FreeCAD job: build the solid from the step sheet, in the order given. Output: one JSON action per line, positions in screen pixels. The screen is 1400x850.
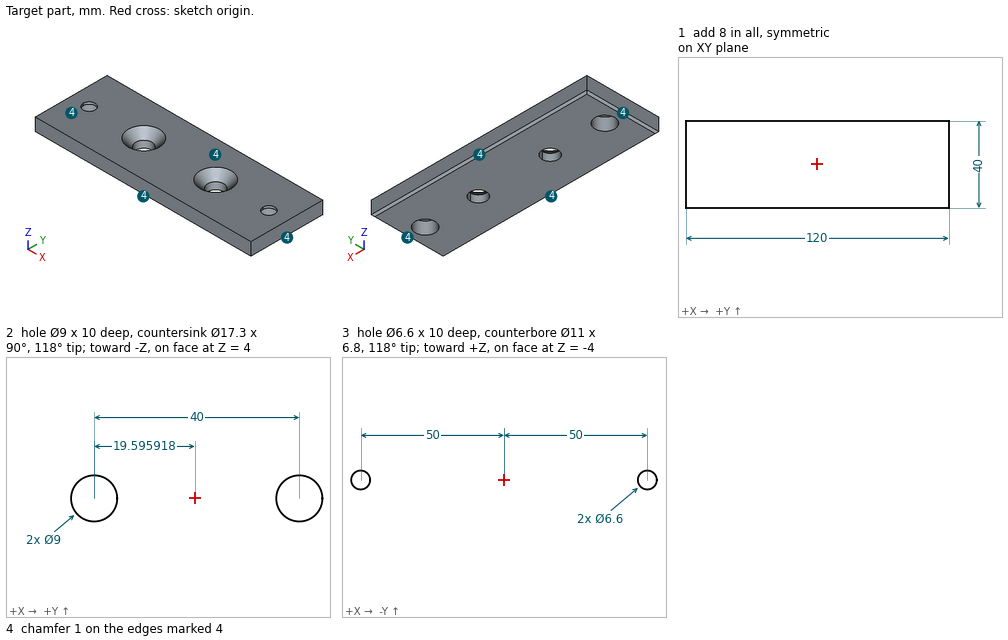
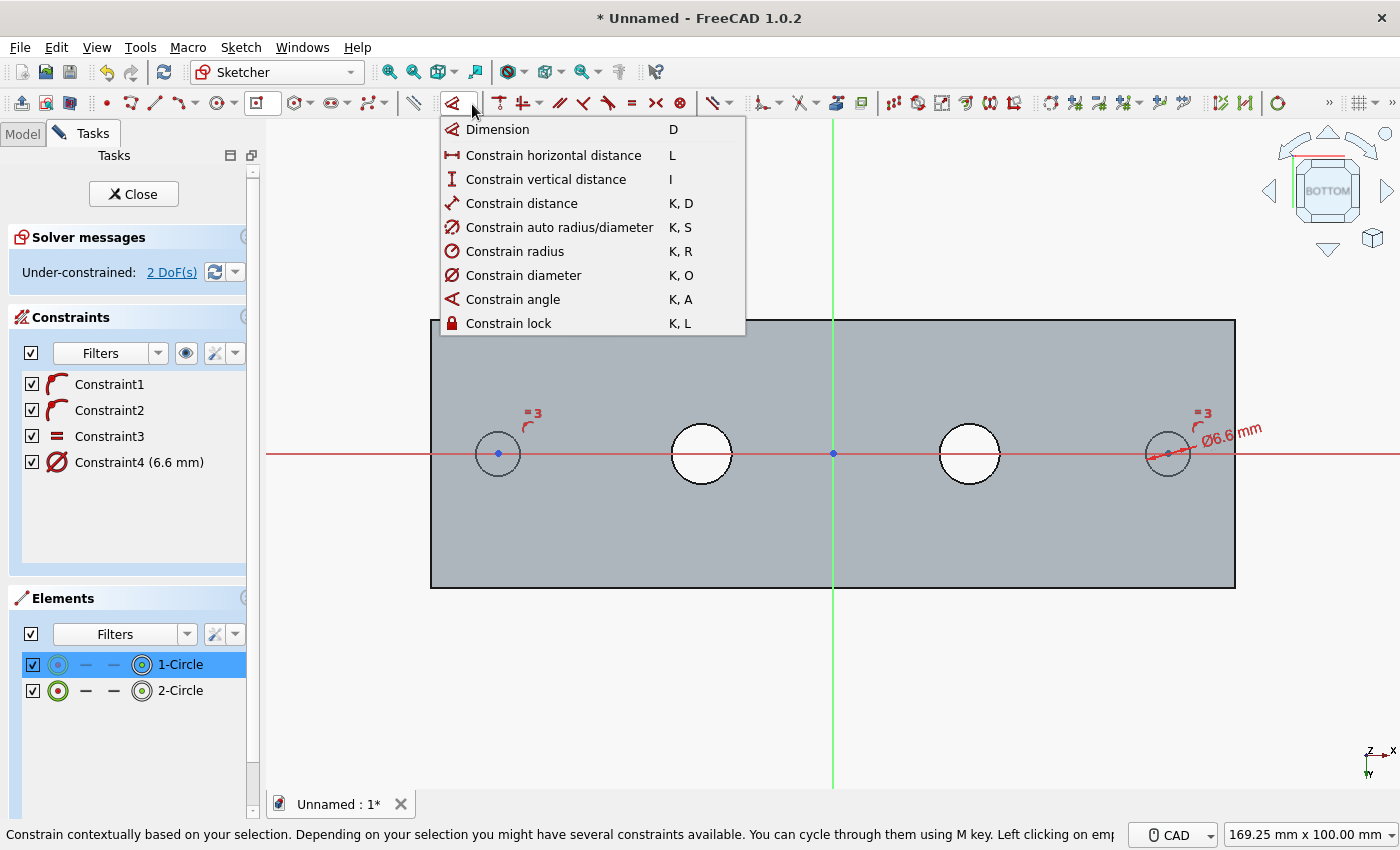
{"action": "left_click", "coordinate": [593, 155]}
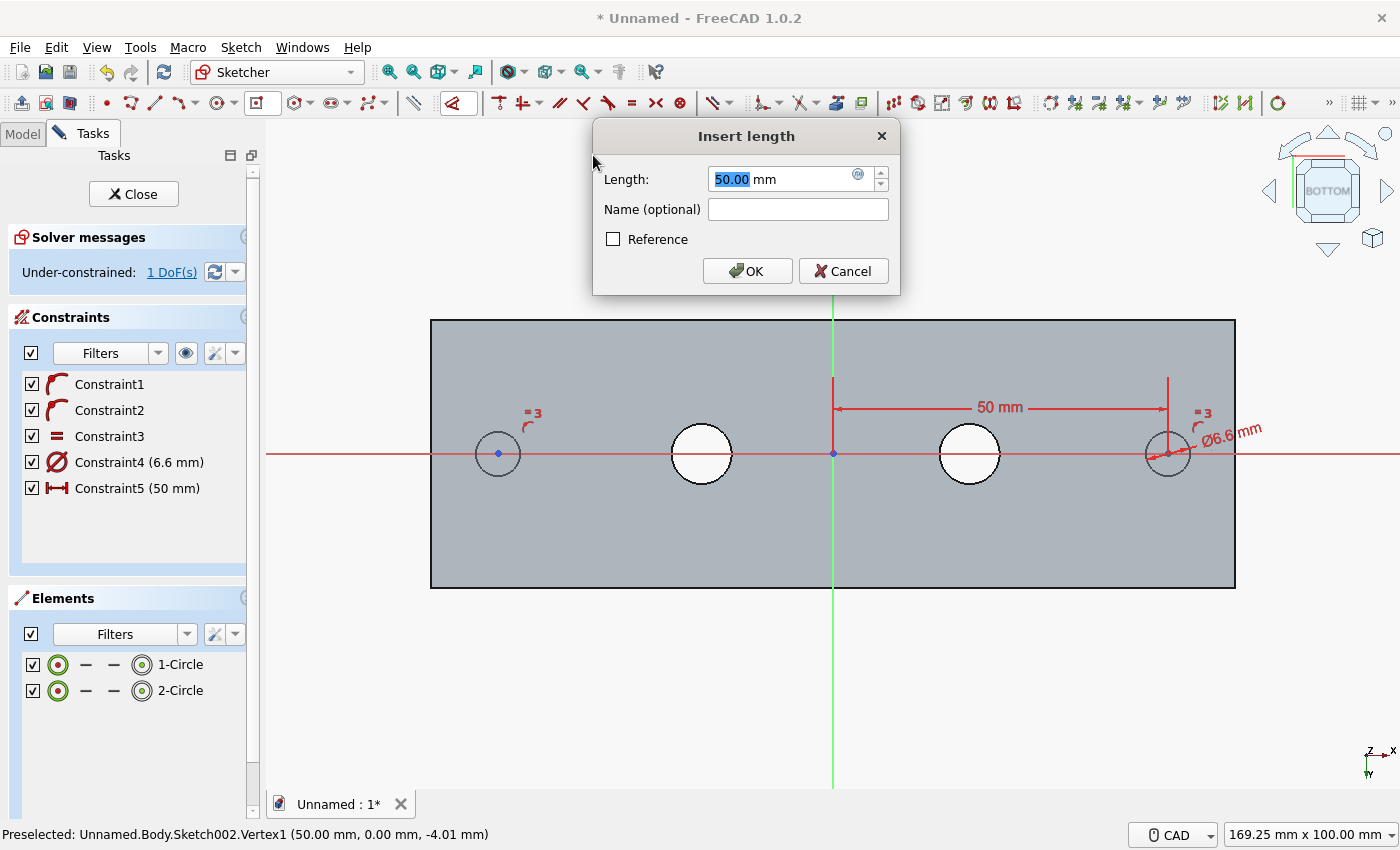
{"action": "type", "text": "50"}
{"action": "key", "text": "Return"}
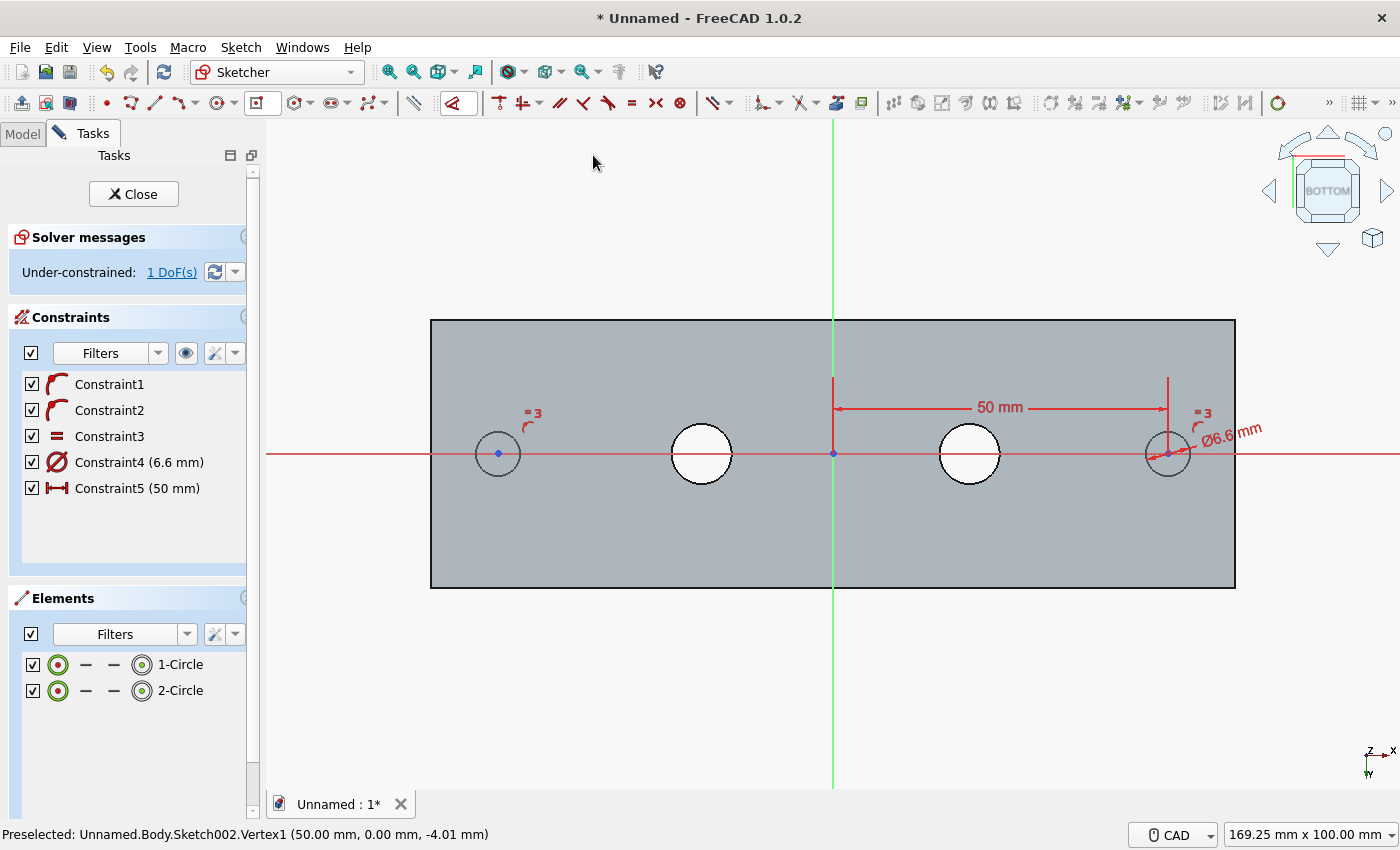
{"action": "left_click", "coordinate": [498, 454]}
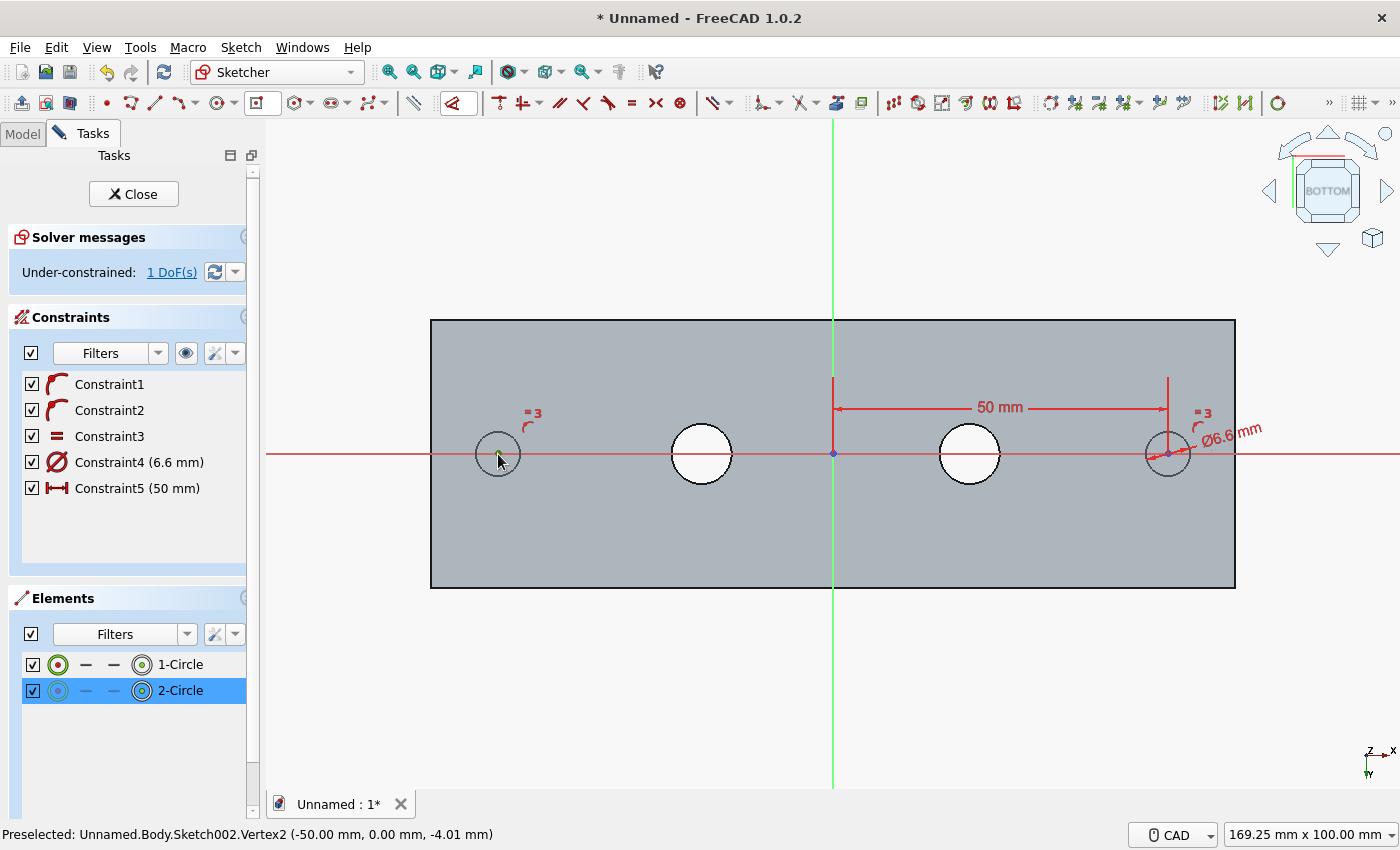
{"action": "key", "text": "l"}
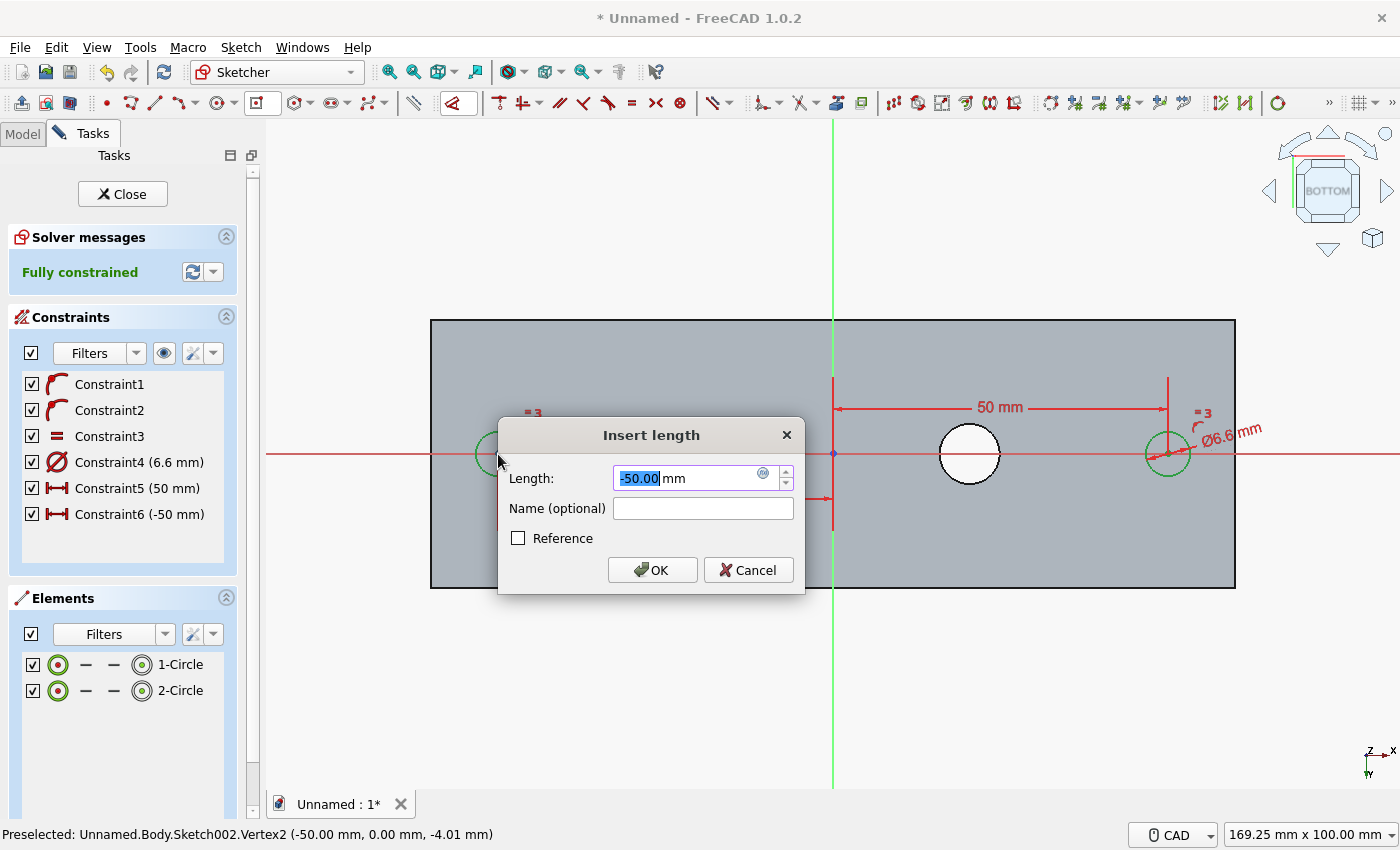
{"action": "type", "text": "-50"}
{"action": "key", "text": "Return"}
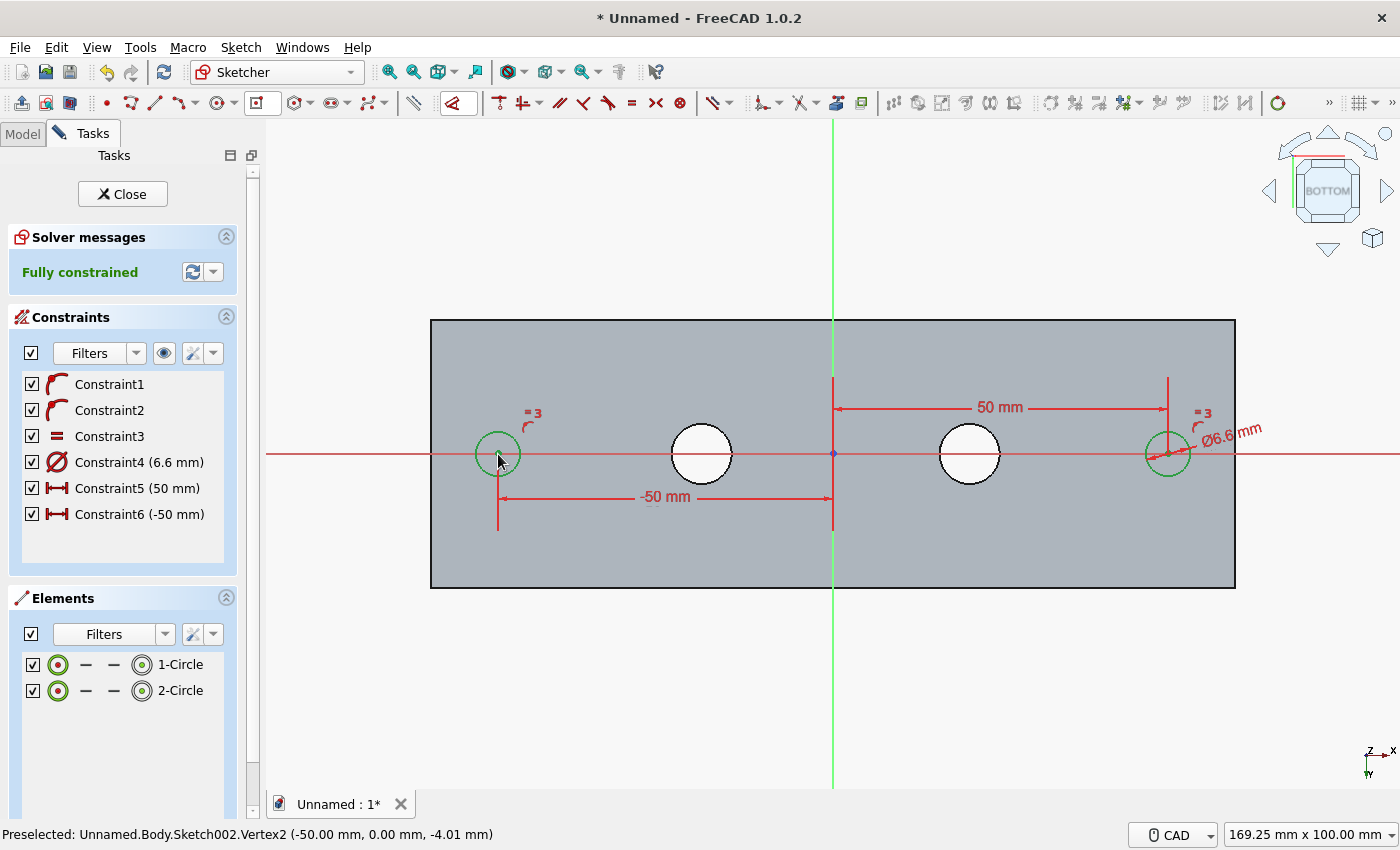
{"action": "left_click", "coordinate": [123, 194]}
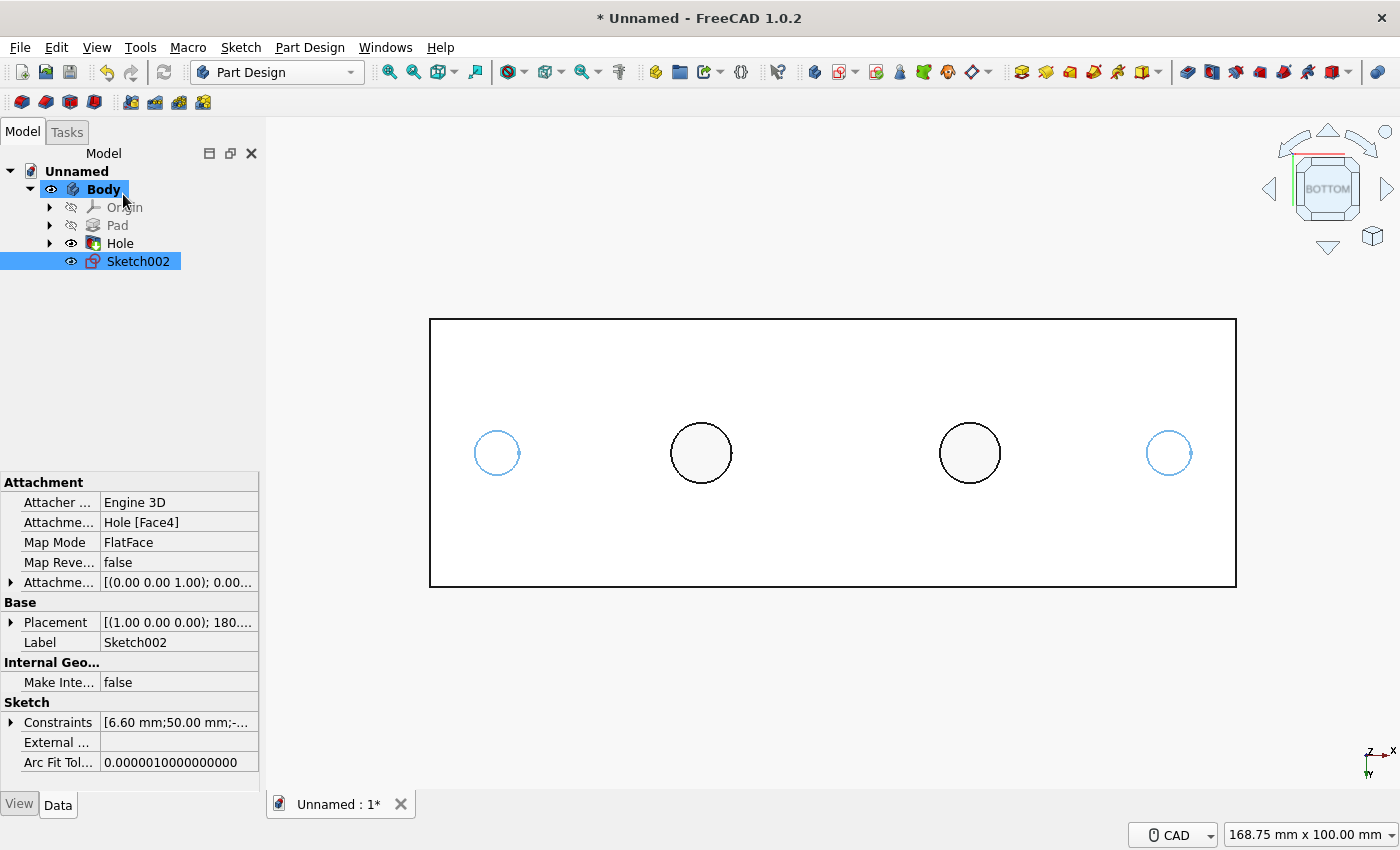
{"action": "left_click", "coordinate": [1212, 72]}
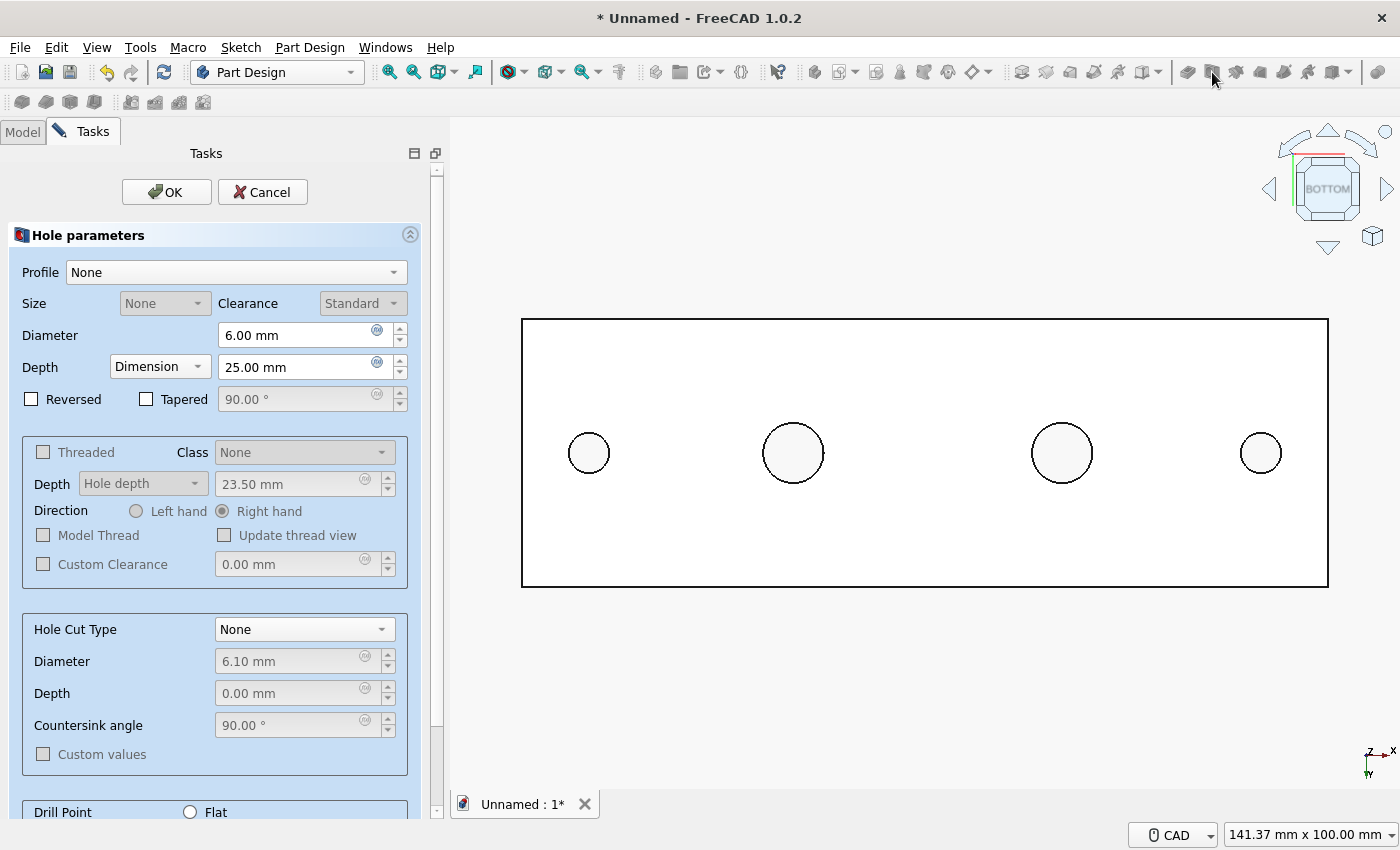
{"action": "triple_click", "coordinate": [305, 335]}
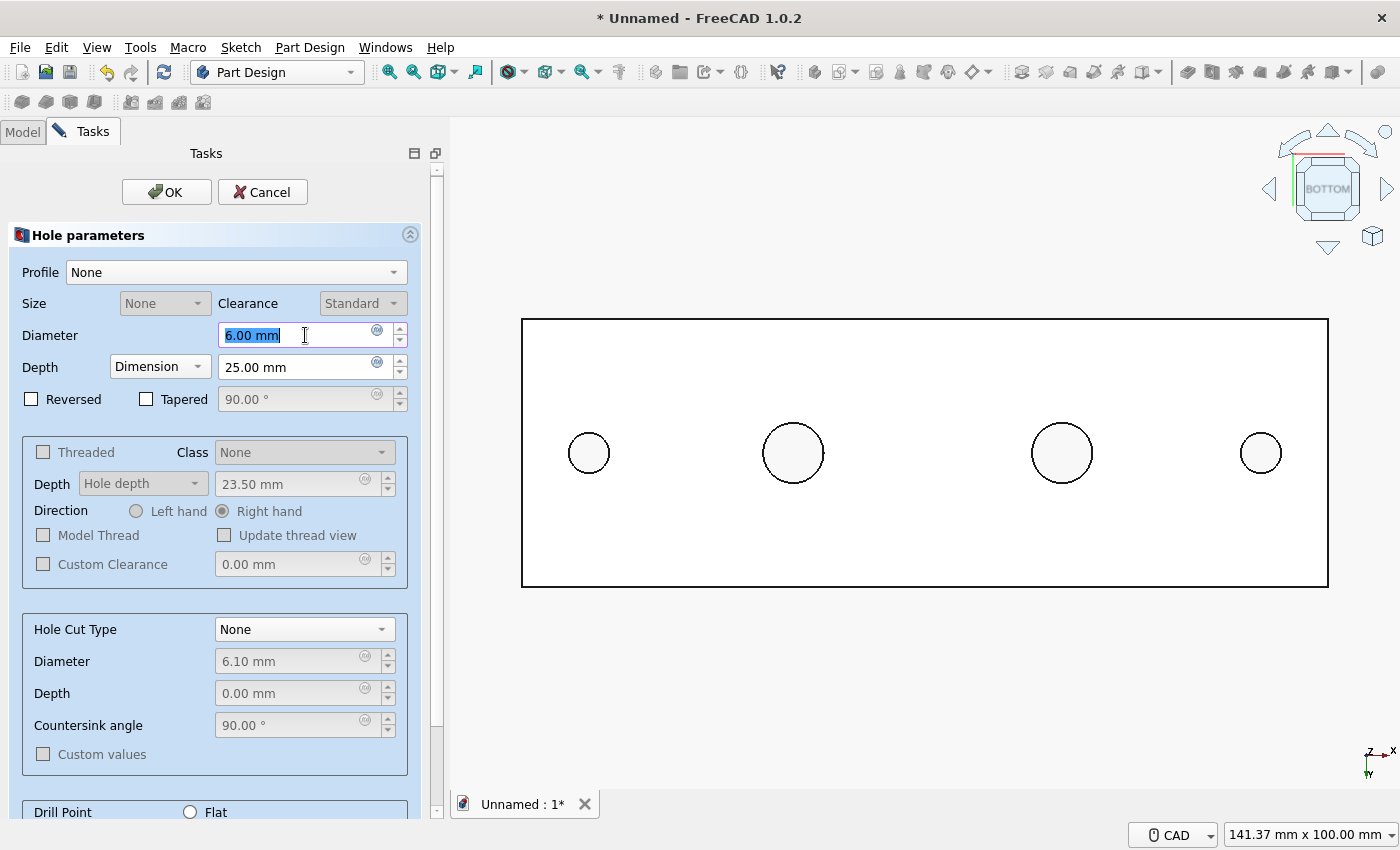
{"action": "type", "text": "6.6"}
{"action": "key", "text": "Tab"}